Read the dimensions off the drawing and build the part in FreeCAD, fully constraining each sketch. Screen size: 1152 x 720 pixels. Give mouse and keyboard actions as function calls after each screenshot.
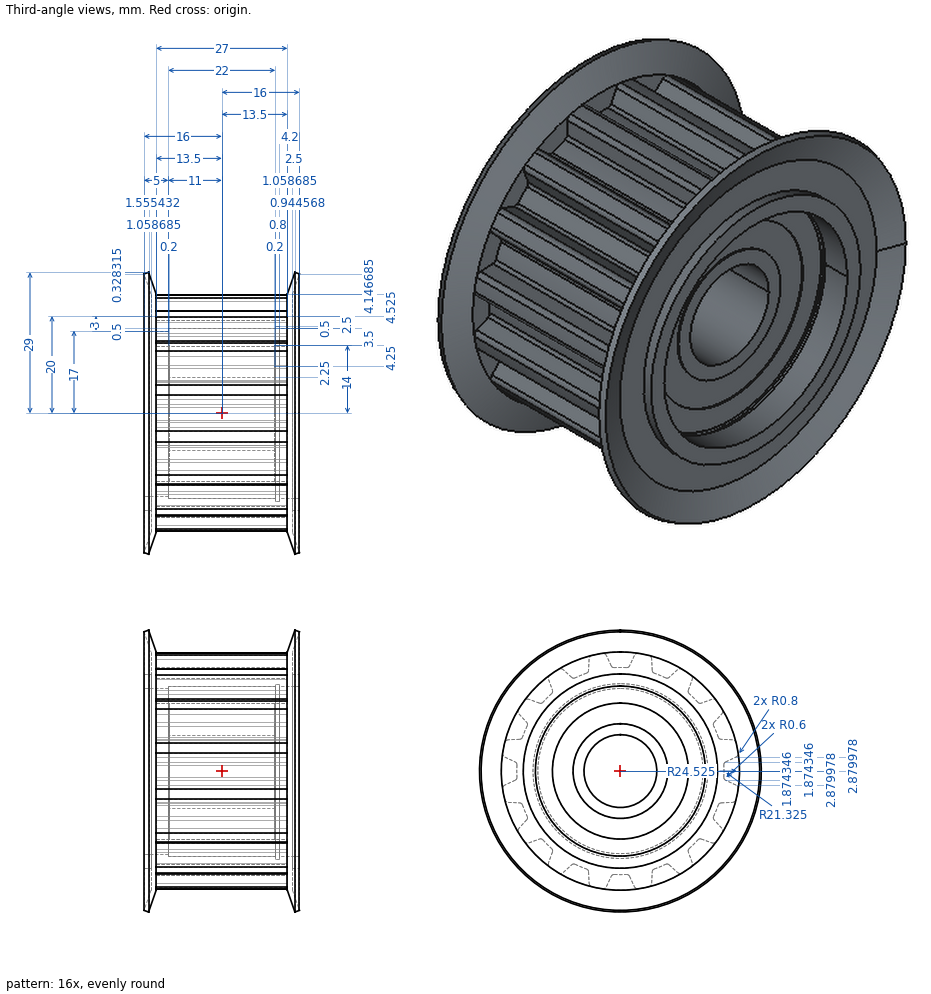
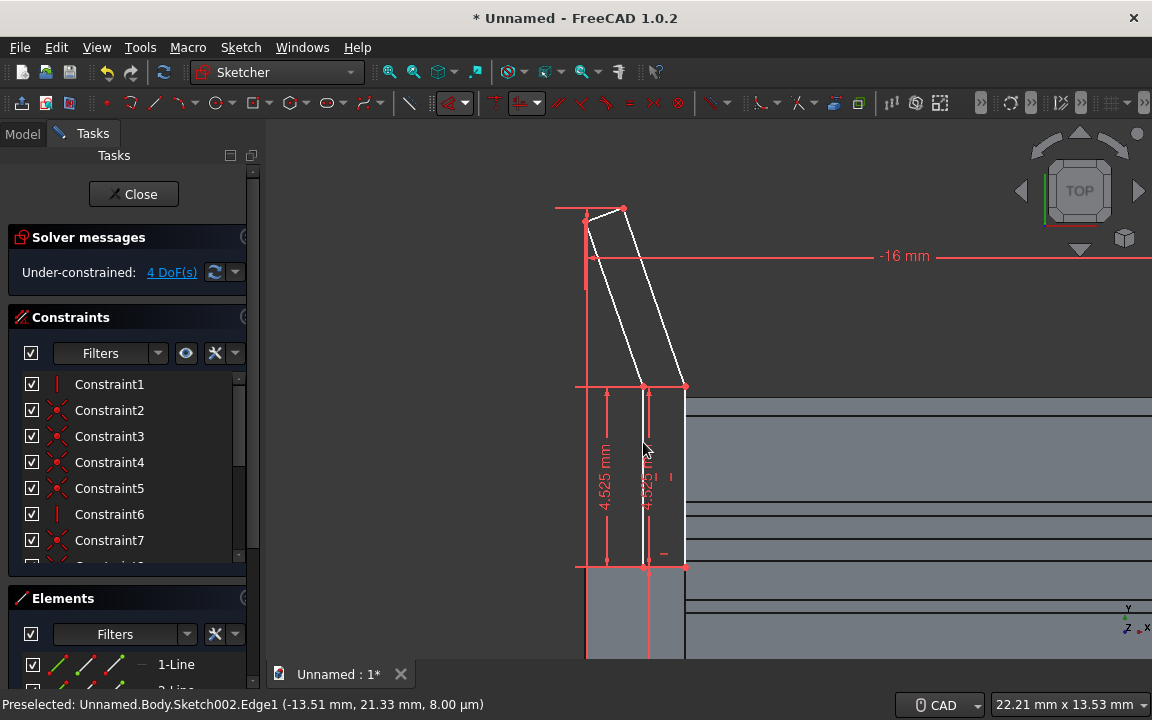
click(685, 567)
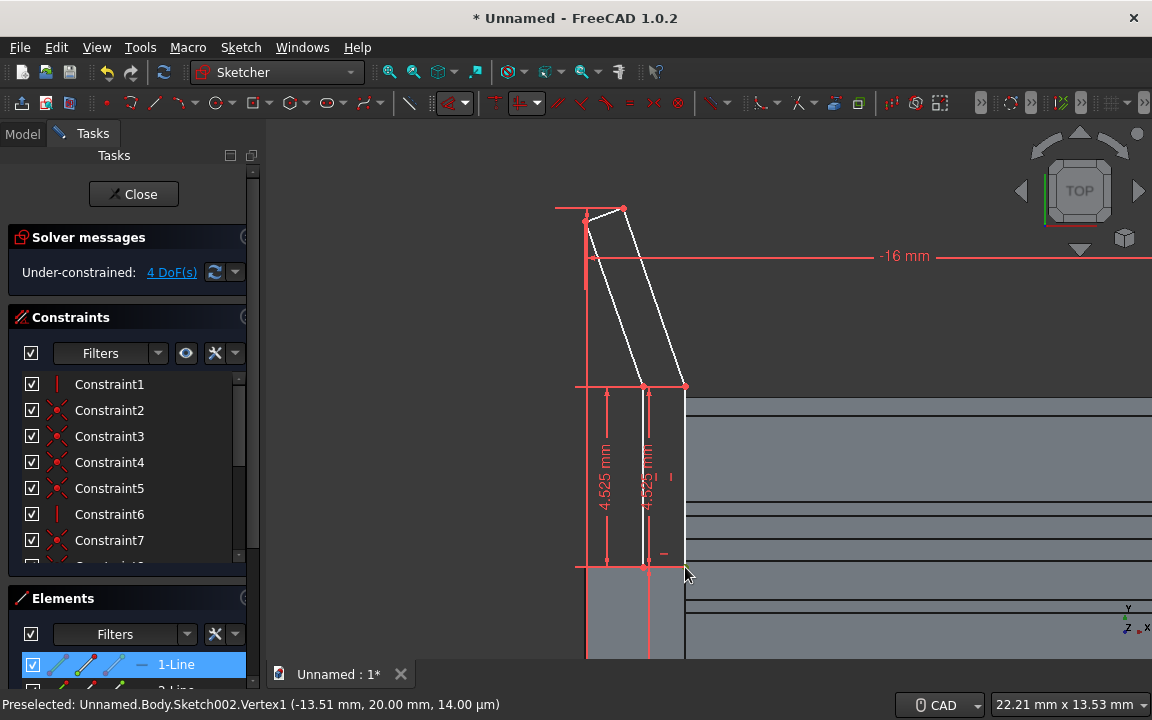
click(468, 104)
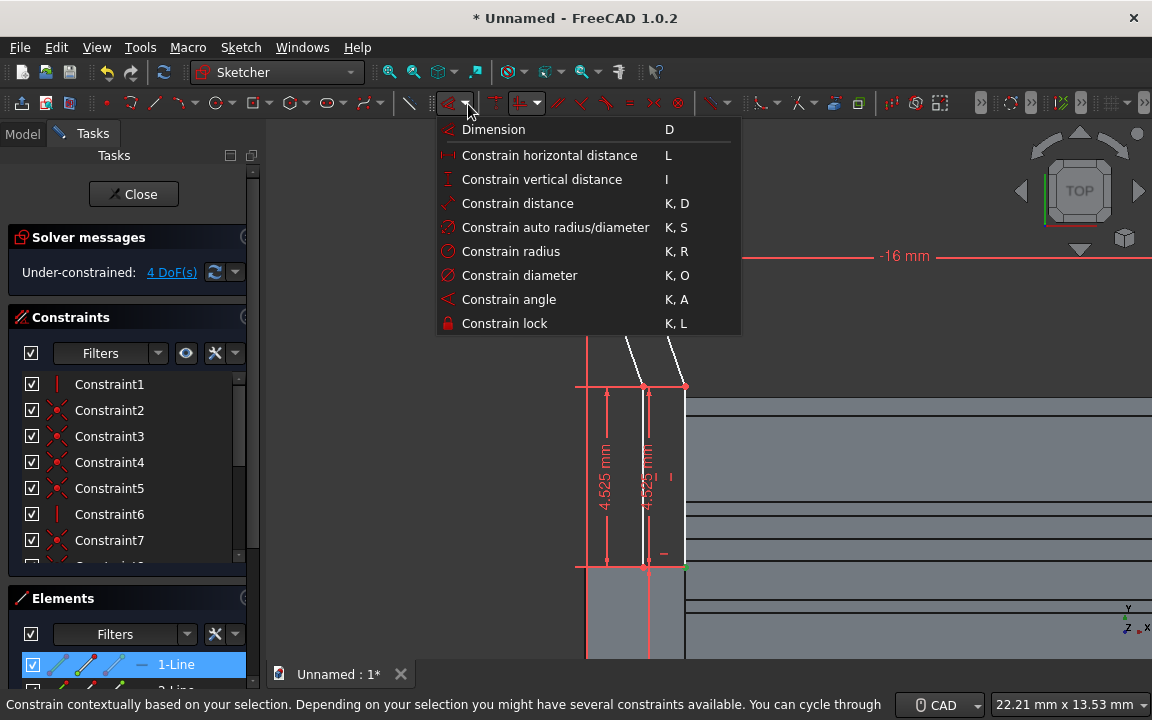
click(589, 155)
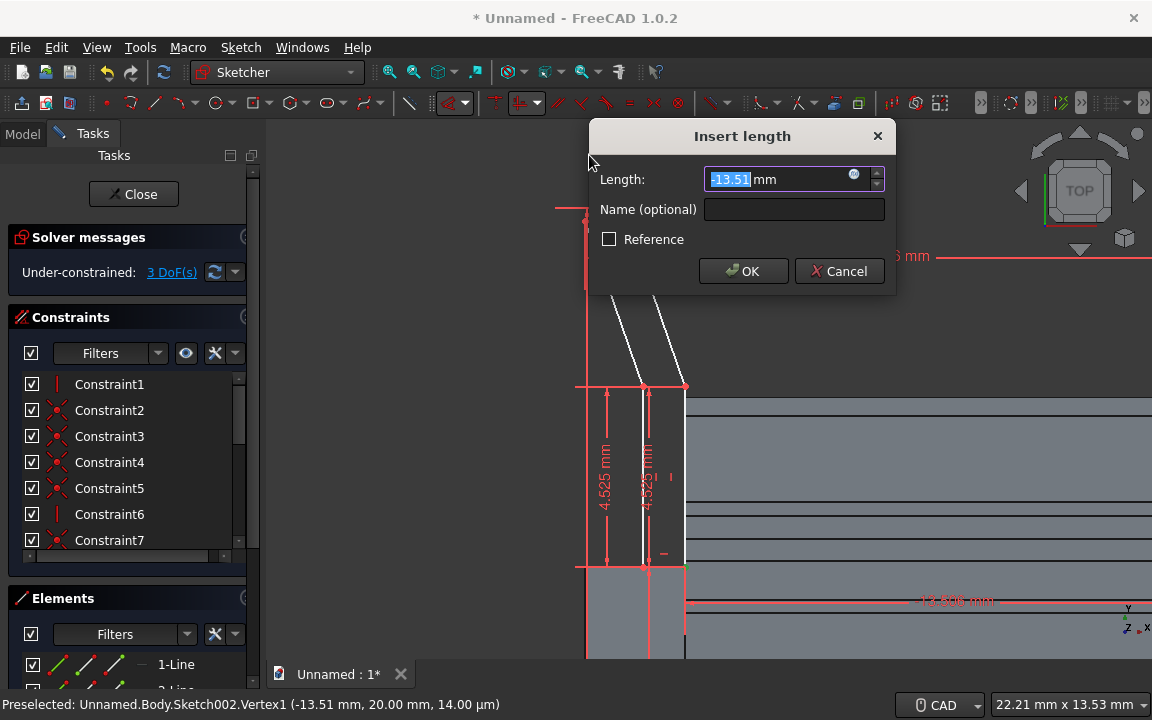
text(-13.5)
key(Return)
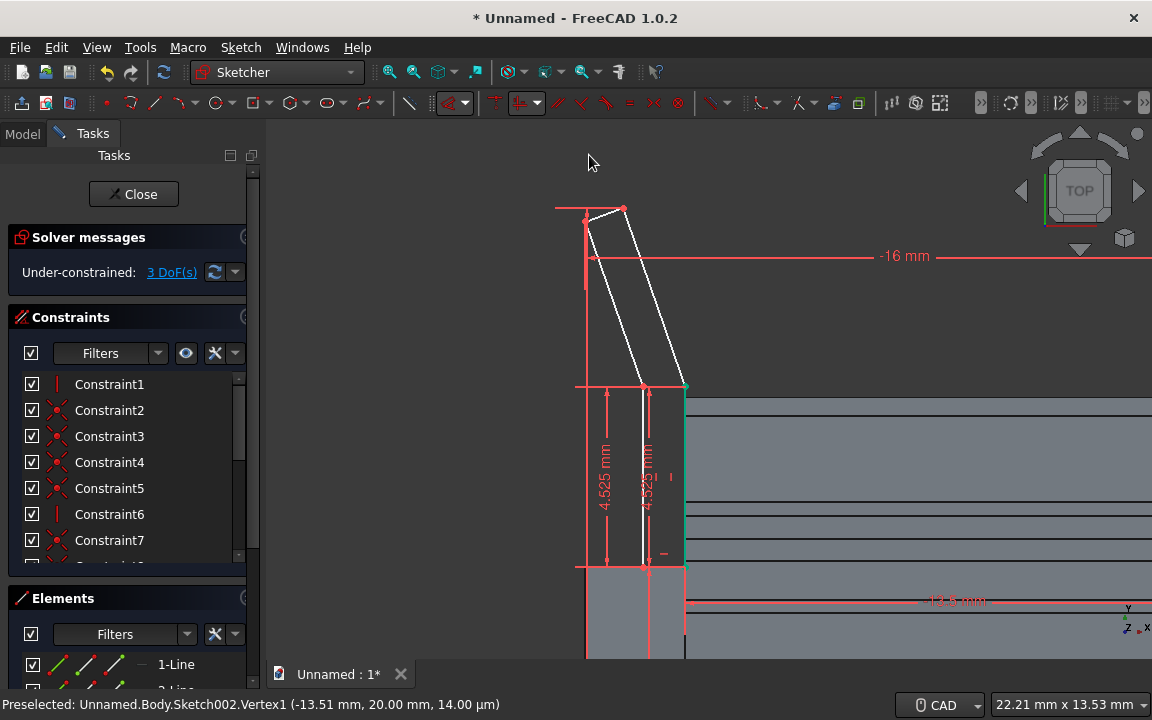
click(656, 567)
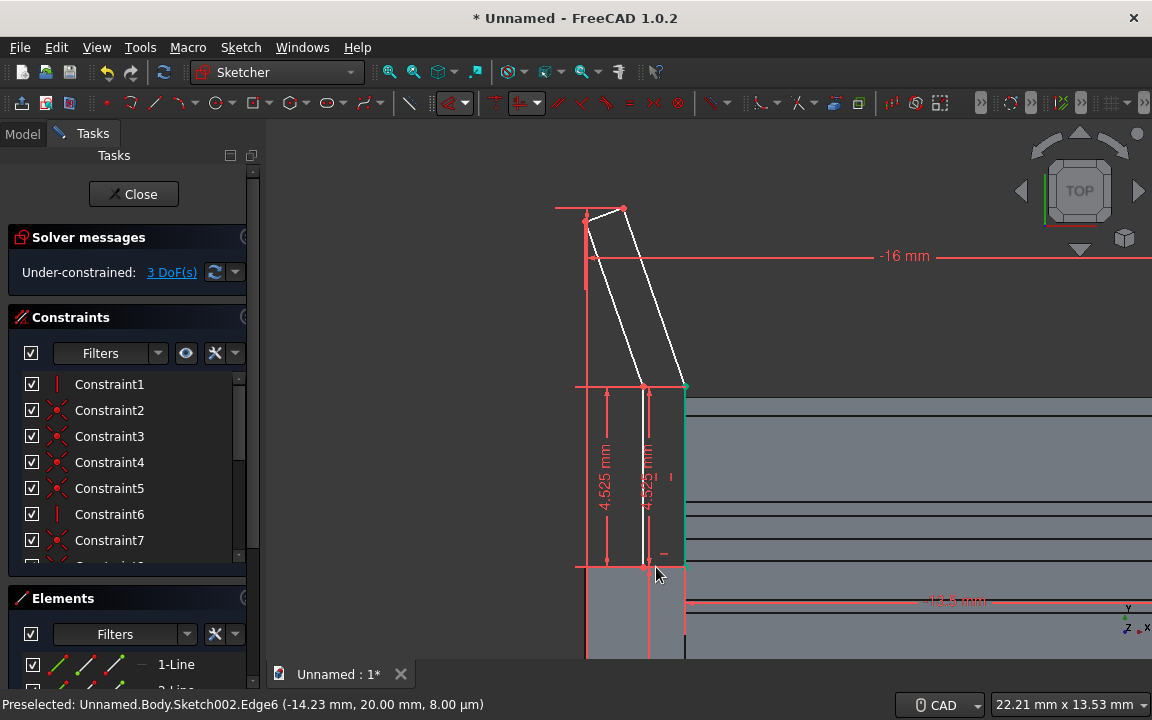
key(l)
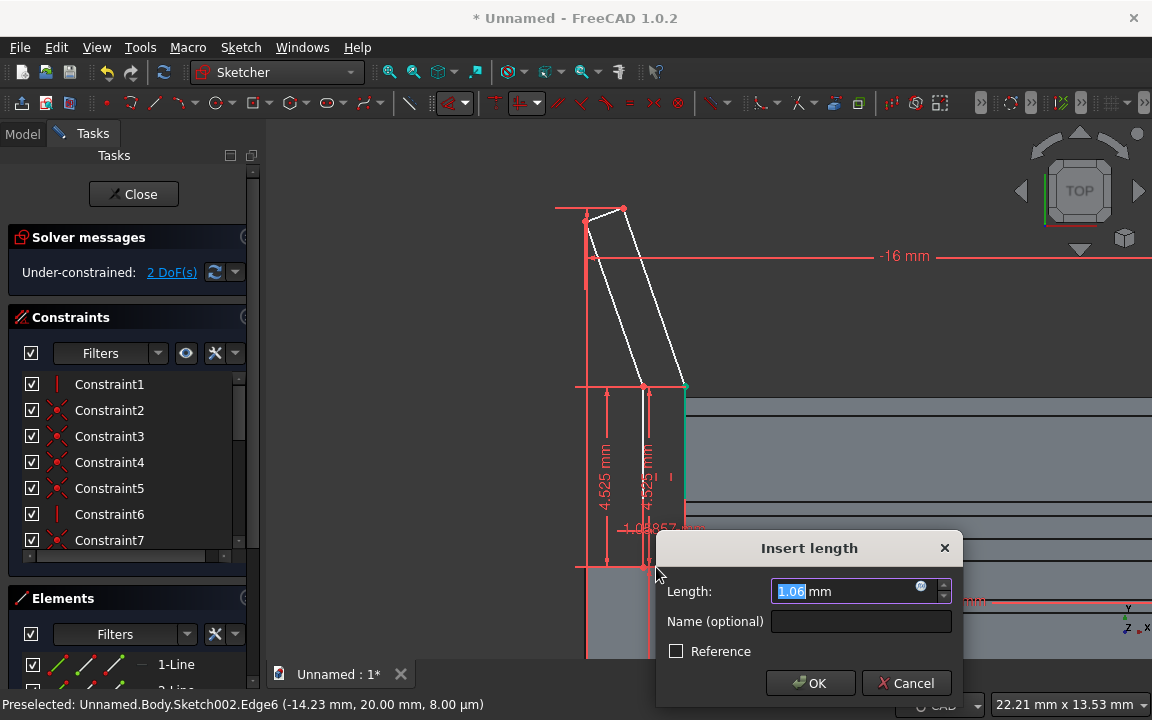
text(1.058685)
key(Return)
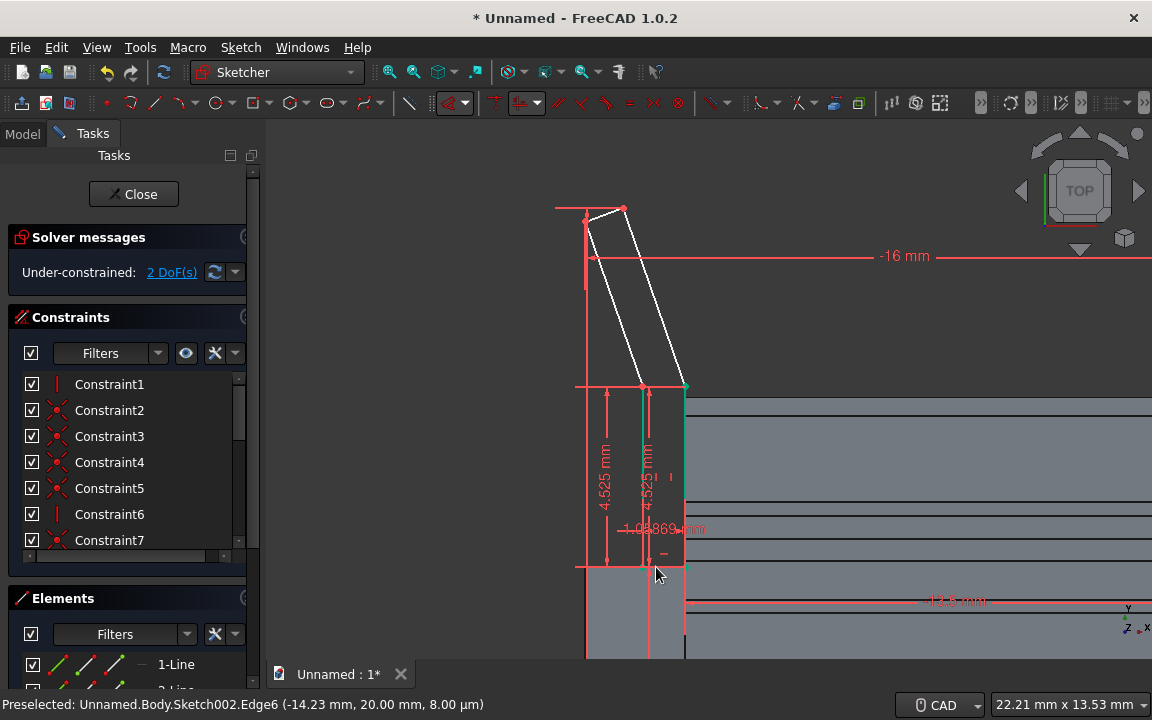
click(667, 333)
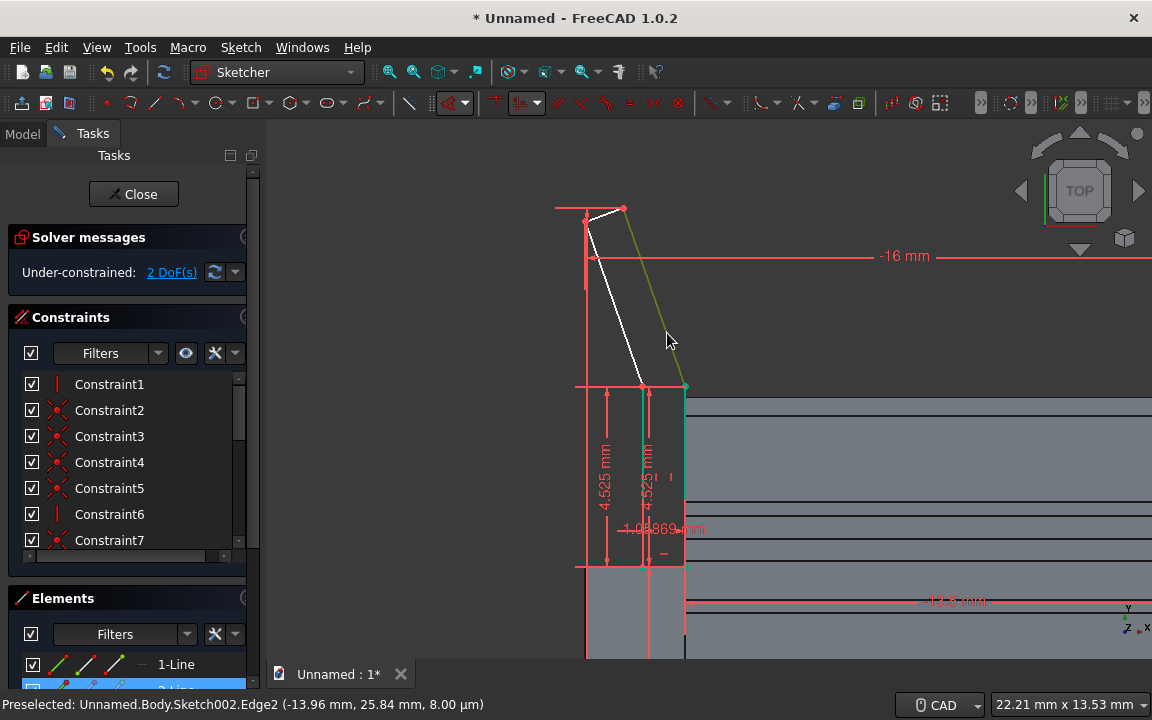
click(468, 104)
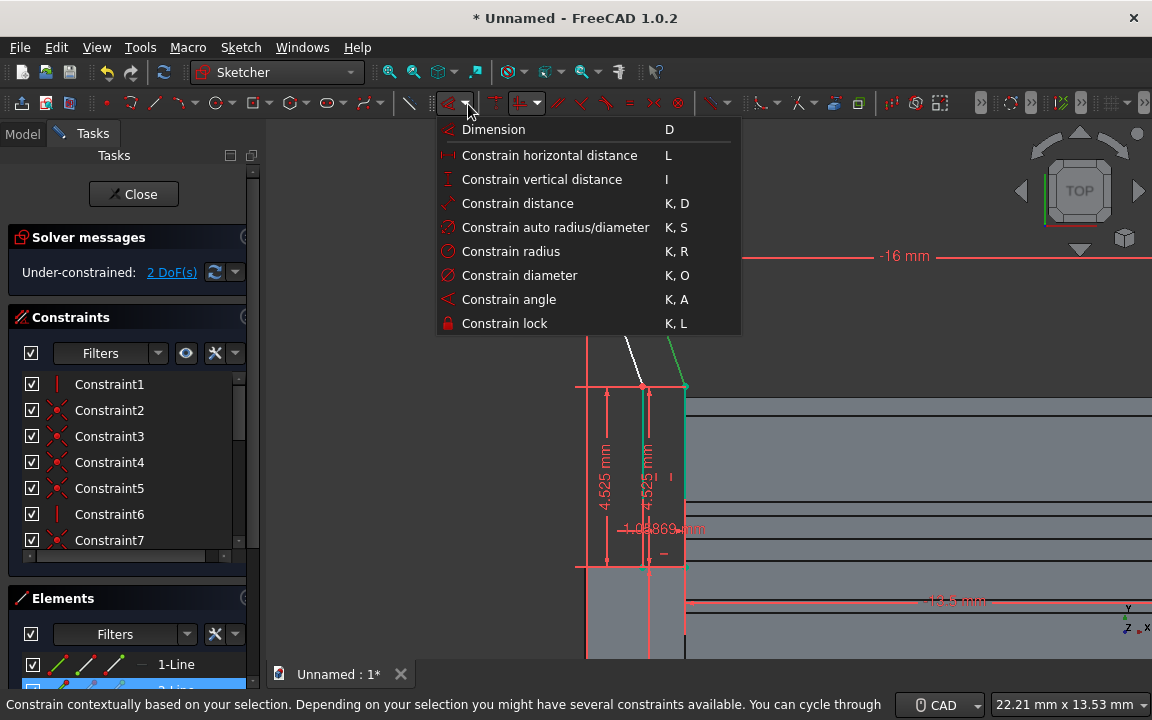
click(589, 155)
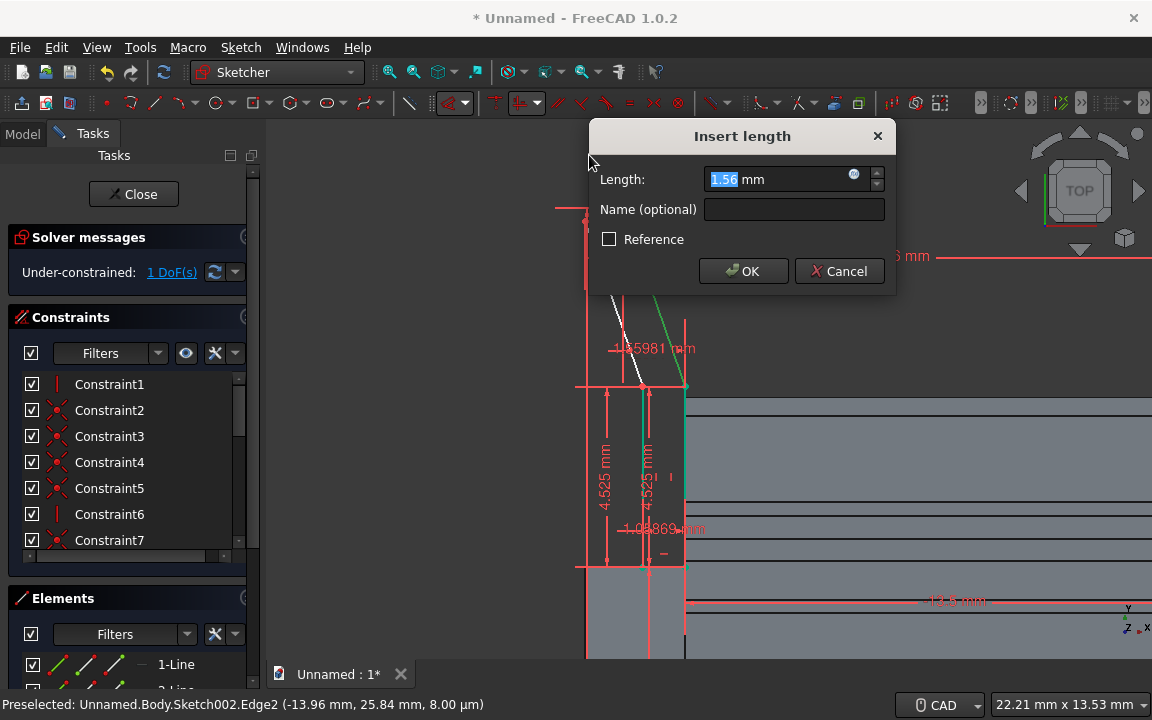
text(1.555432)
key(Return)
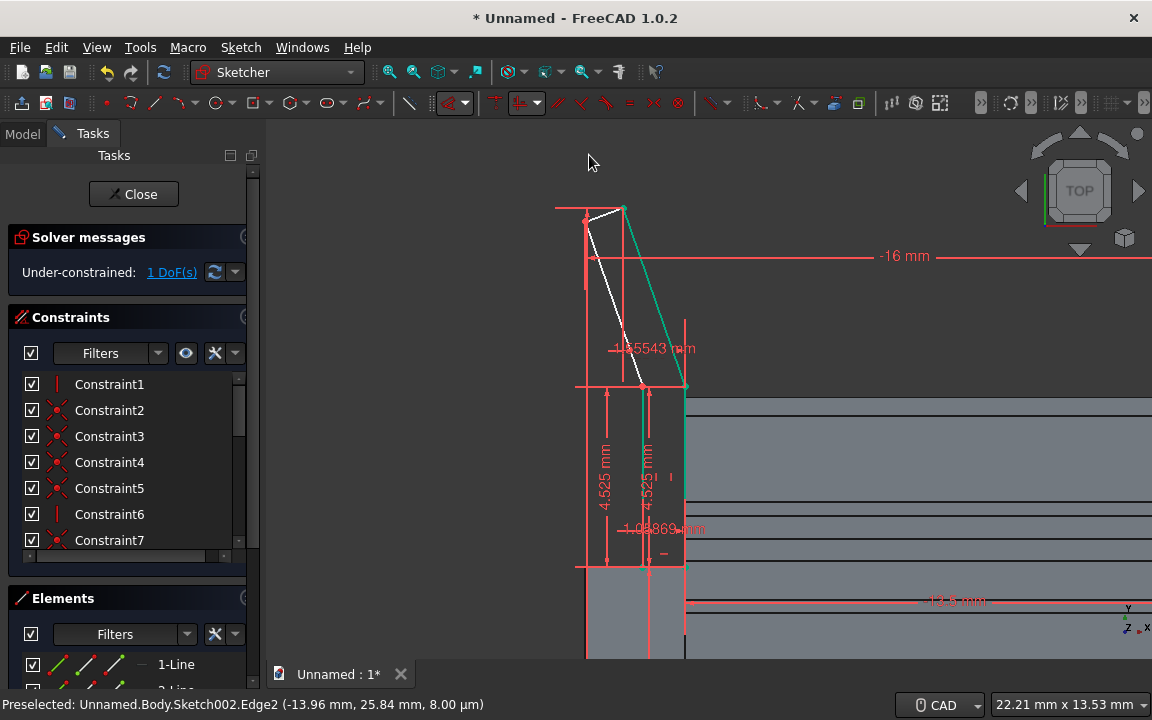
scroll(612, 212, up, 6)